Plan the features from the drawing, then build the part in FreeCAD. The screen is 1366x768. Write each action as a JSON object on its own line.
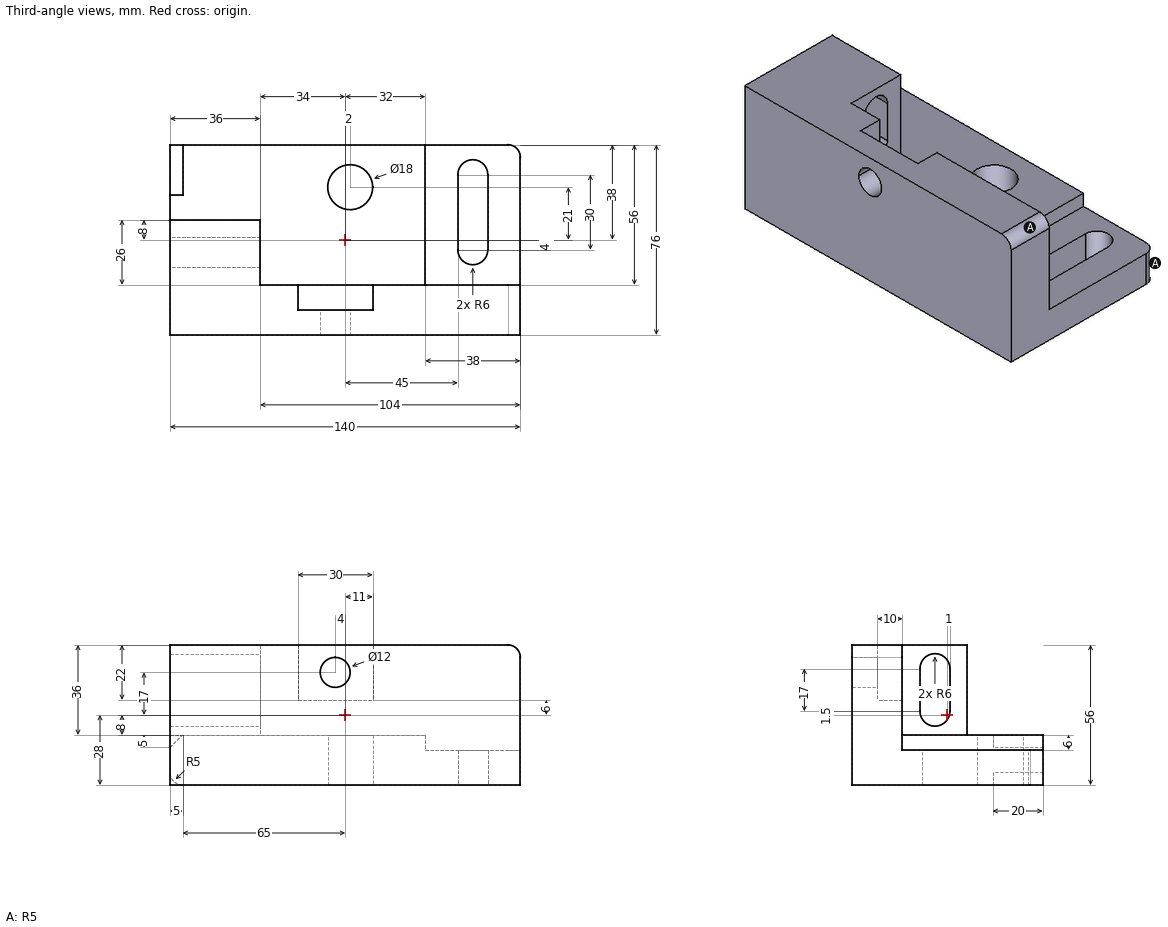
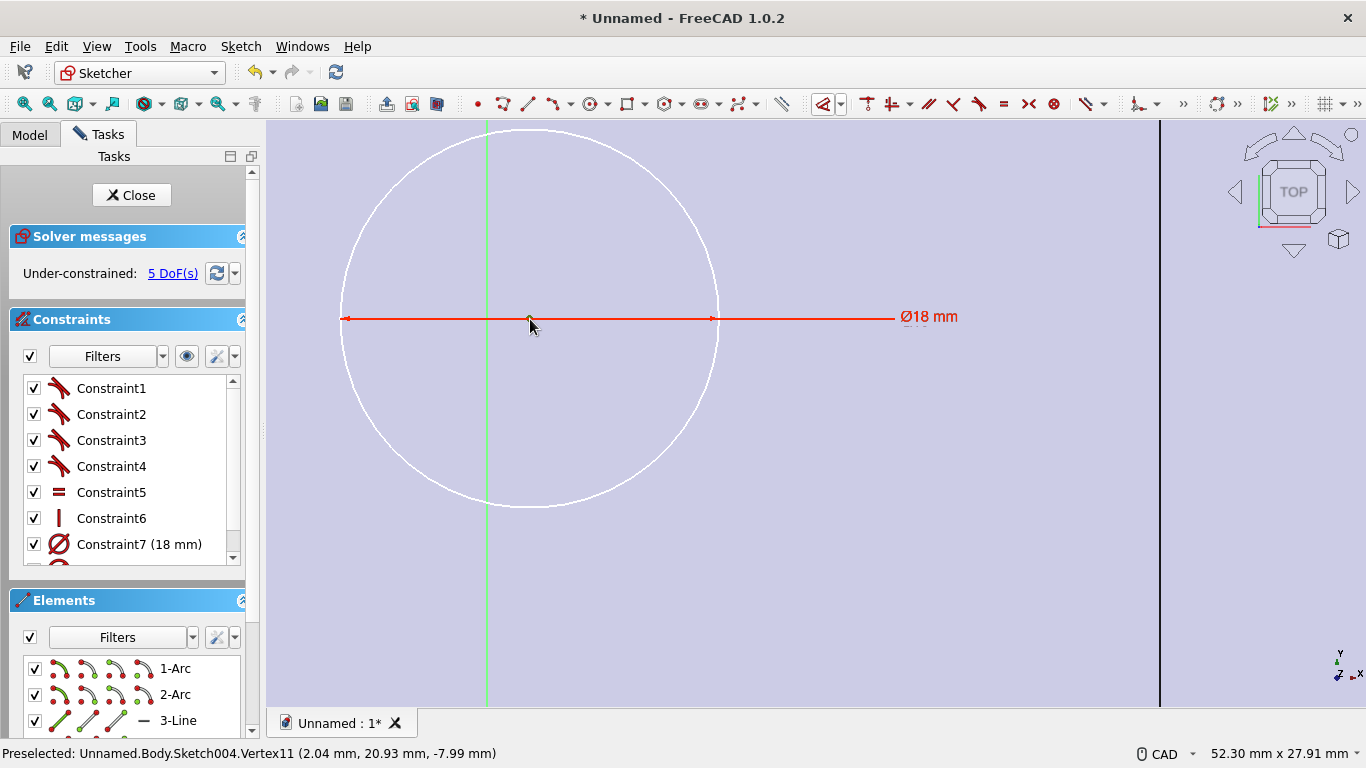
{"action": "key", "text": "l"}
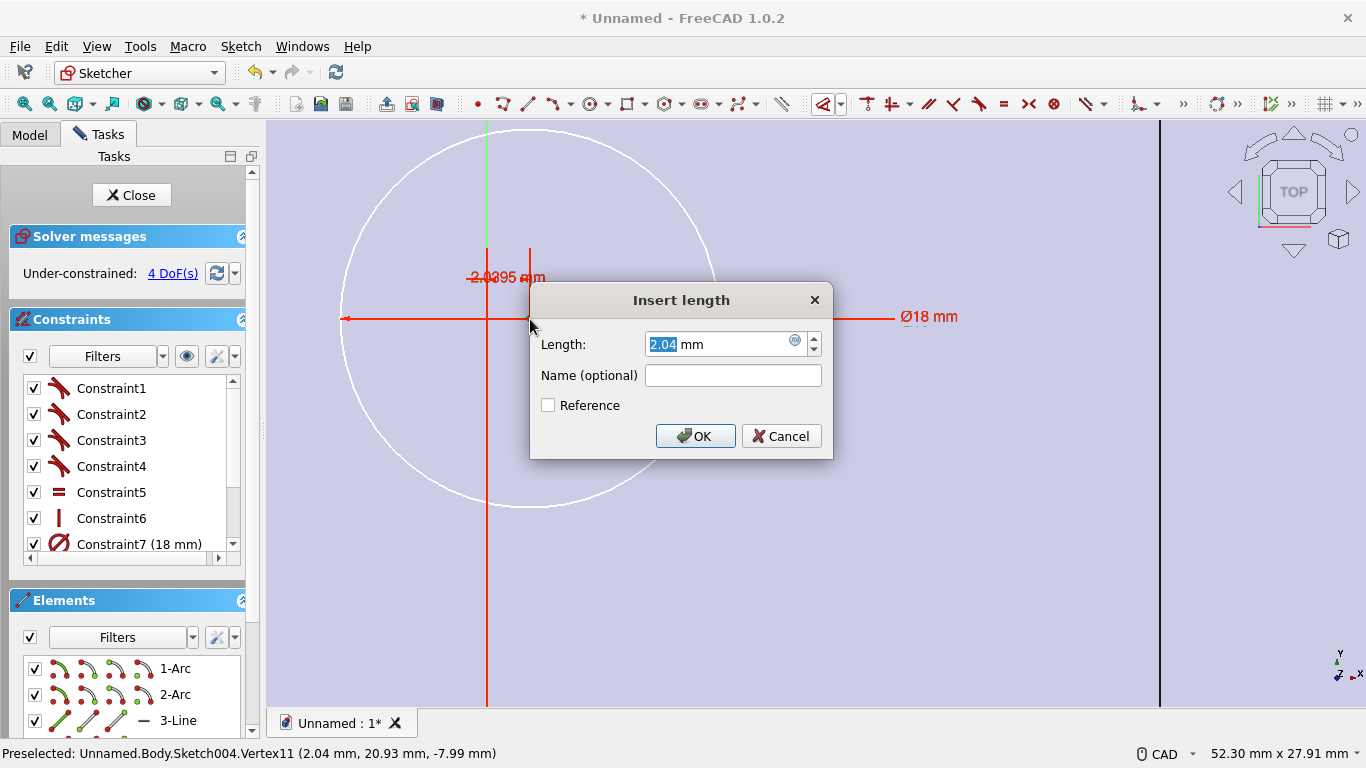
{"action": "type", "text": "2"}
{"action": "key", "text": "Return"}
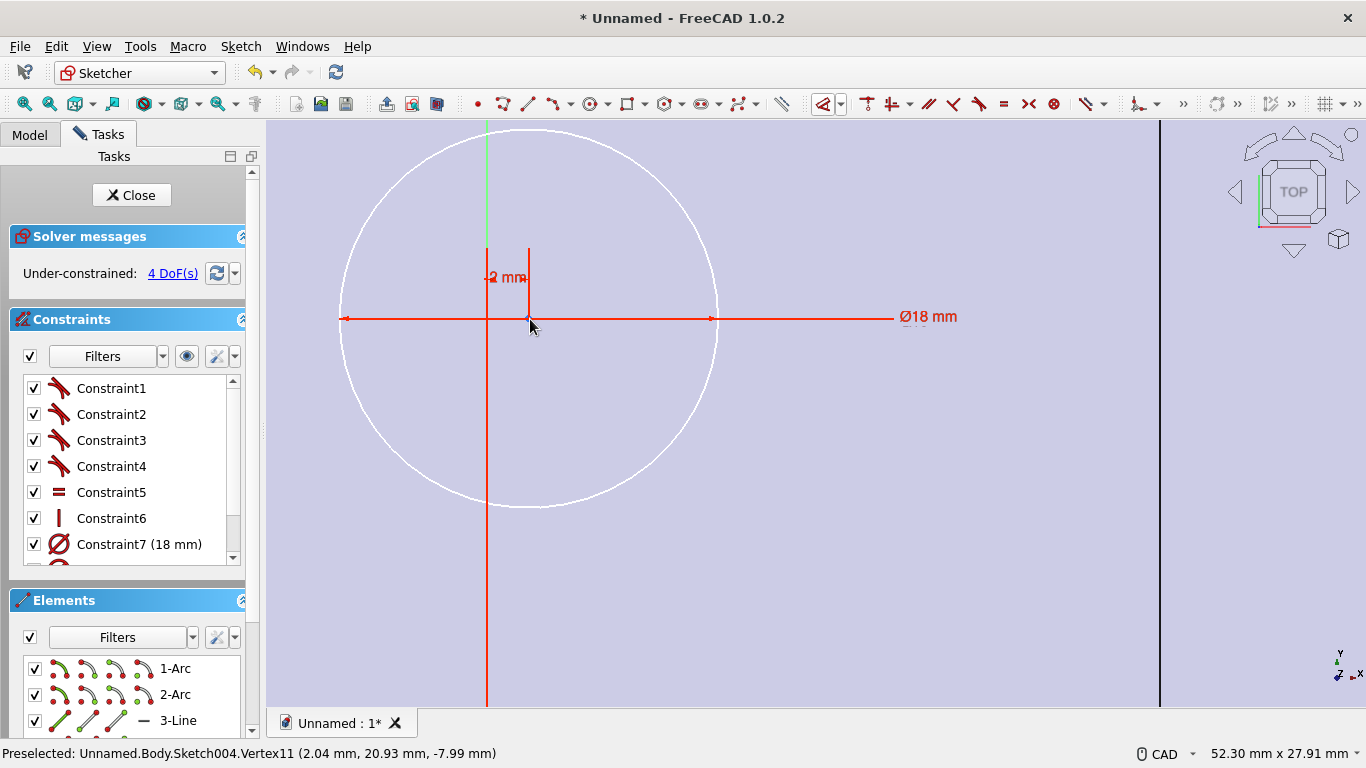
{"action": "scroll", "coordinate": [531, 321], "scroll_direction": "down", "scroll_amount": 4}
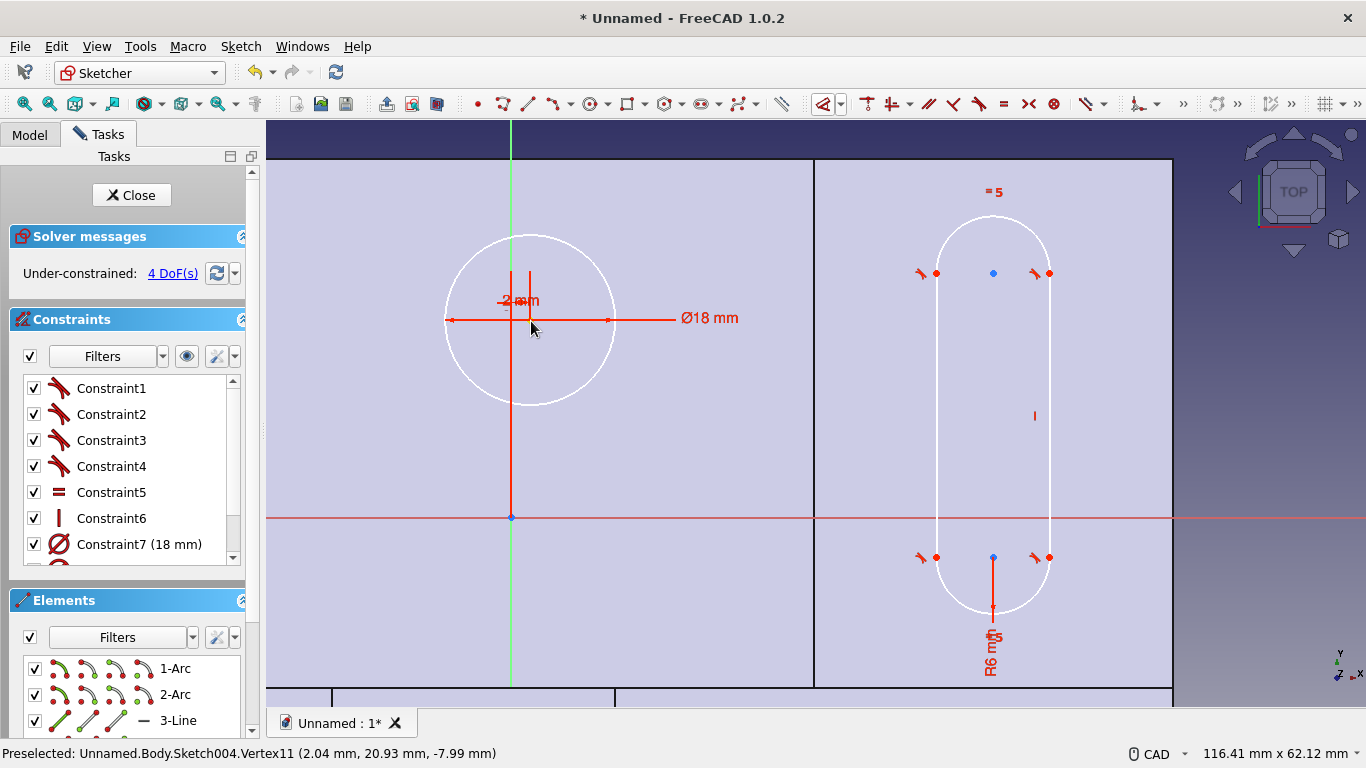
{"action": "left_click", "coordinate": [937, 472]}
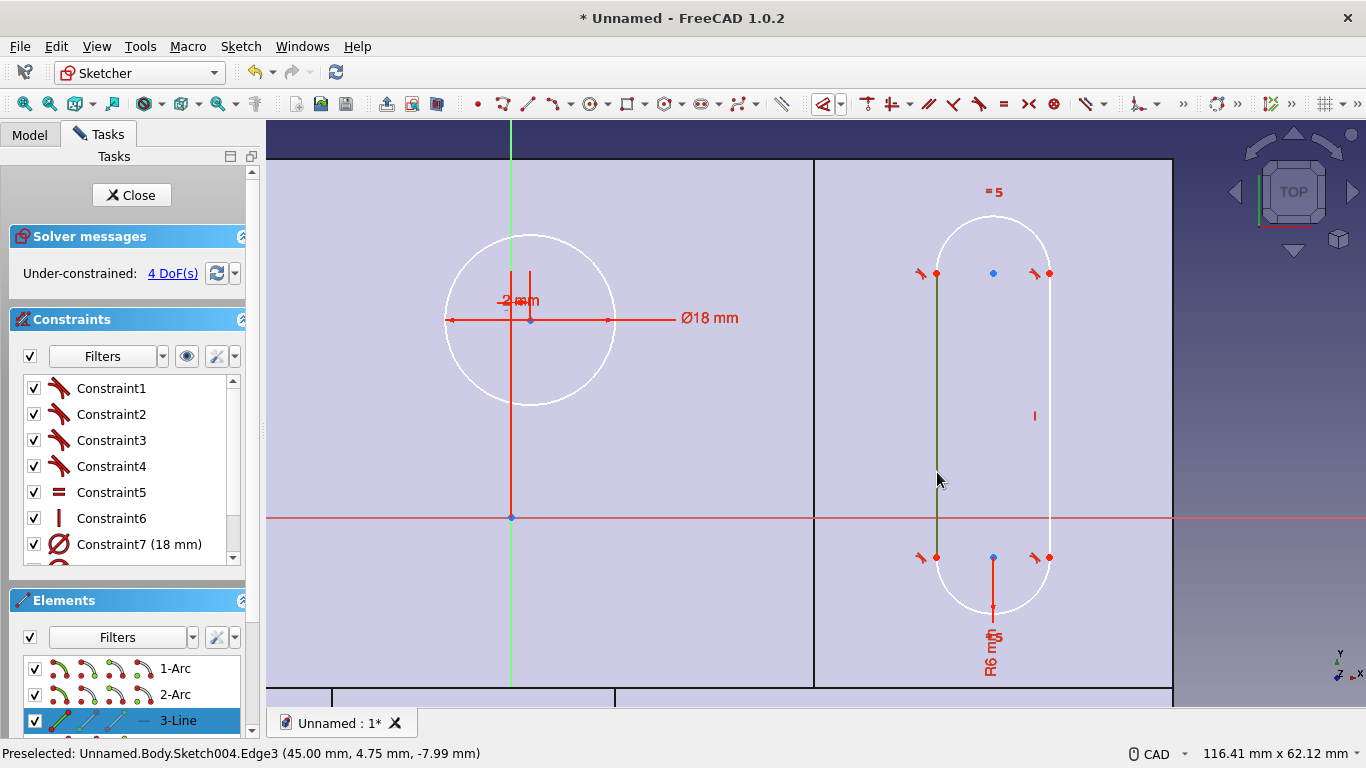
{"action": "left_click", "coordinate": [840, 104]}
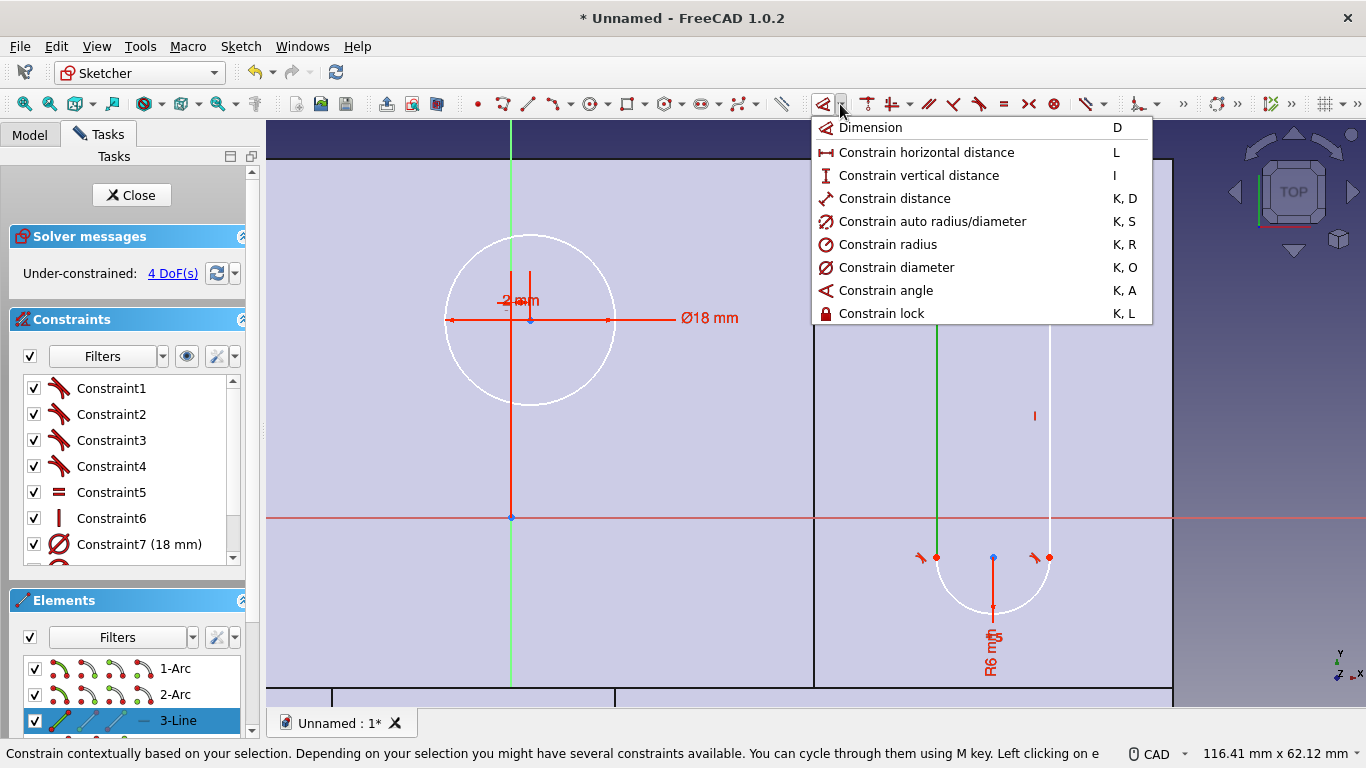
{"action": "left_click", "coordinate": [982, 176]}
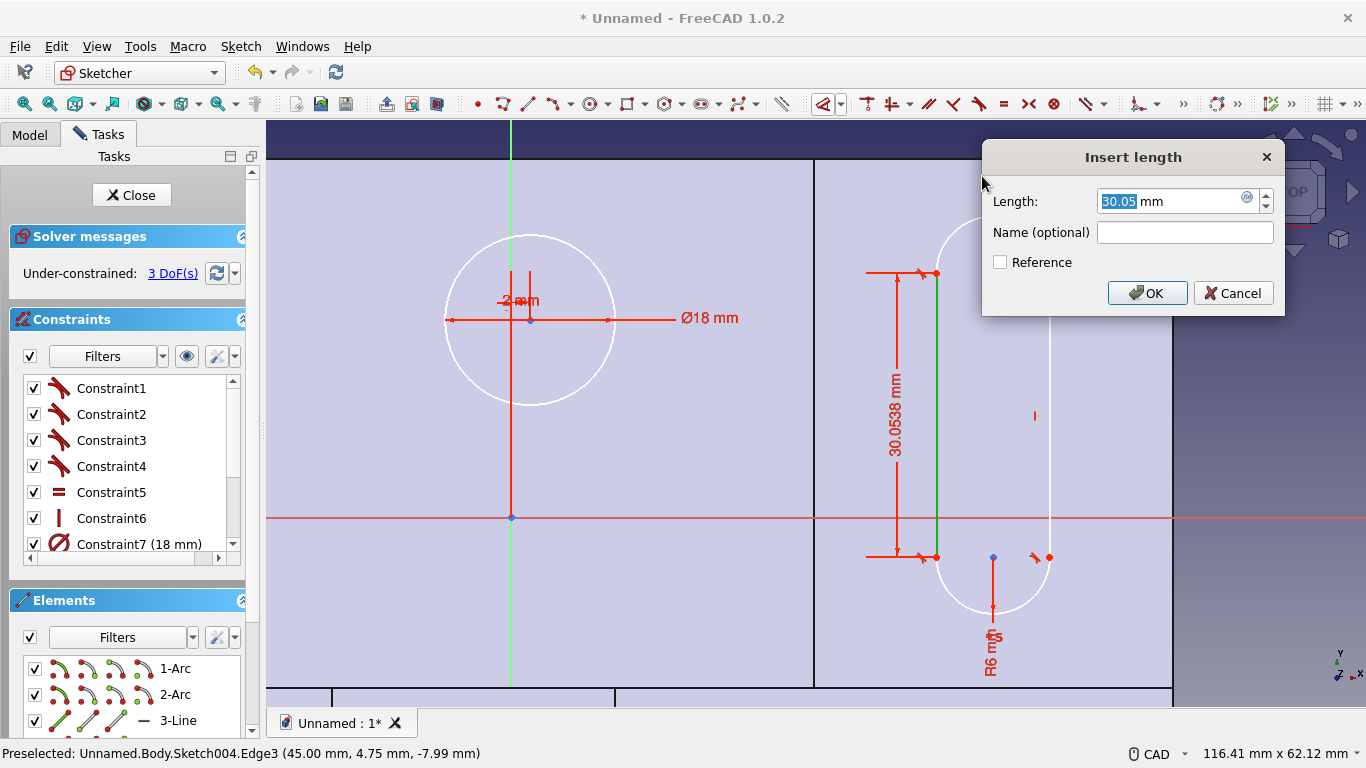
{"action": "type", "text": "30"}
{"action": "key", "text": "Return"}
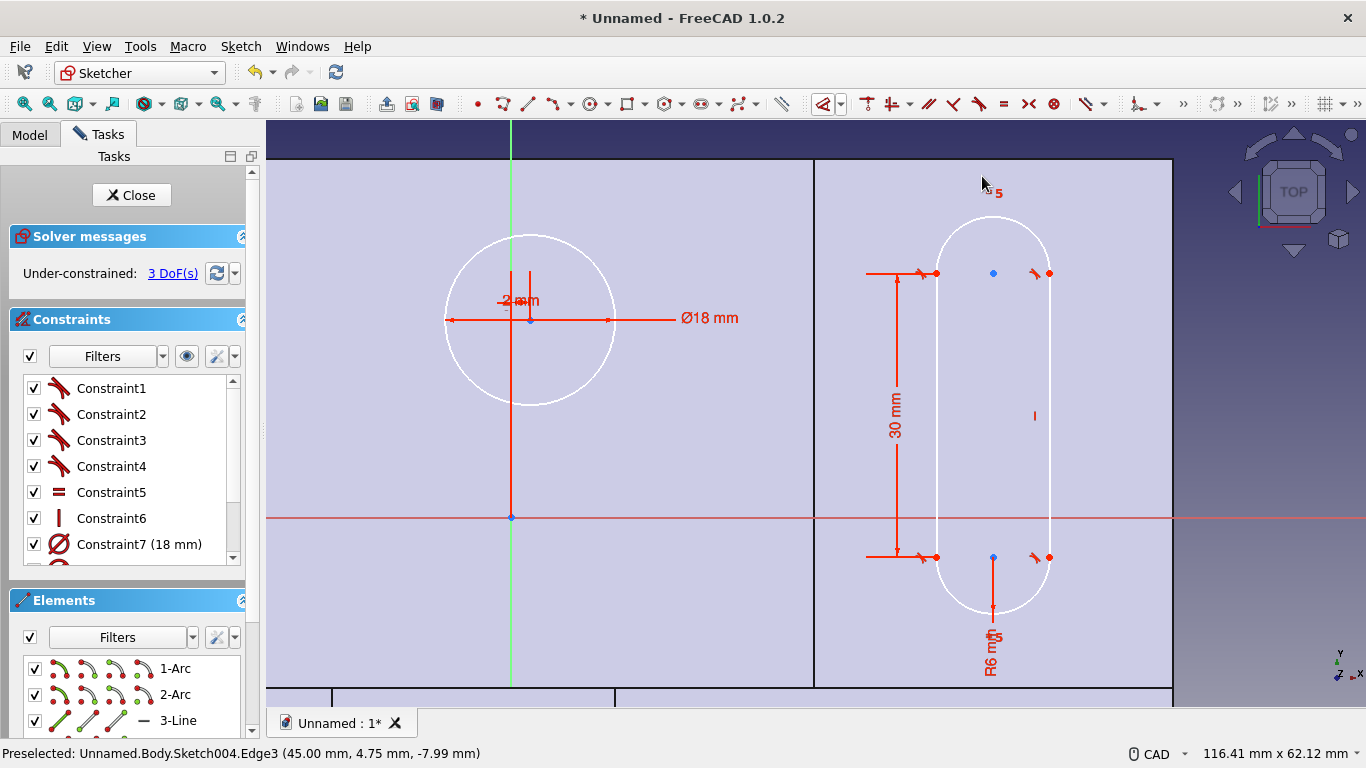
{"action": "left_click", "coordinate": [937, 557]}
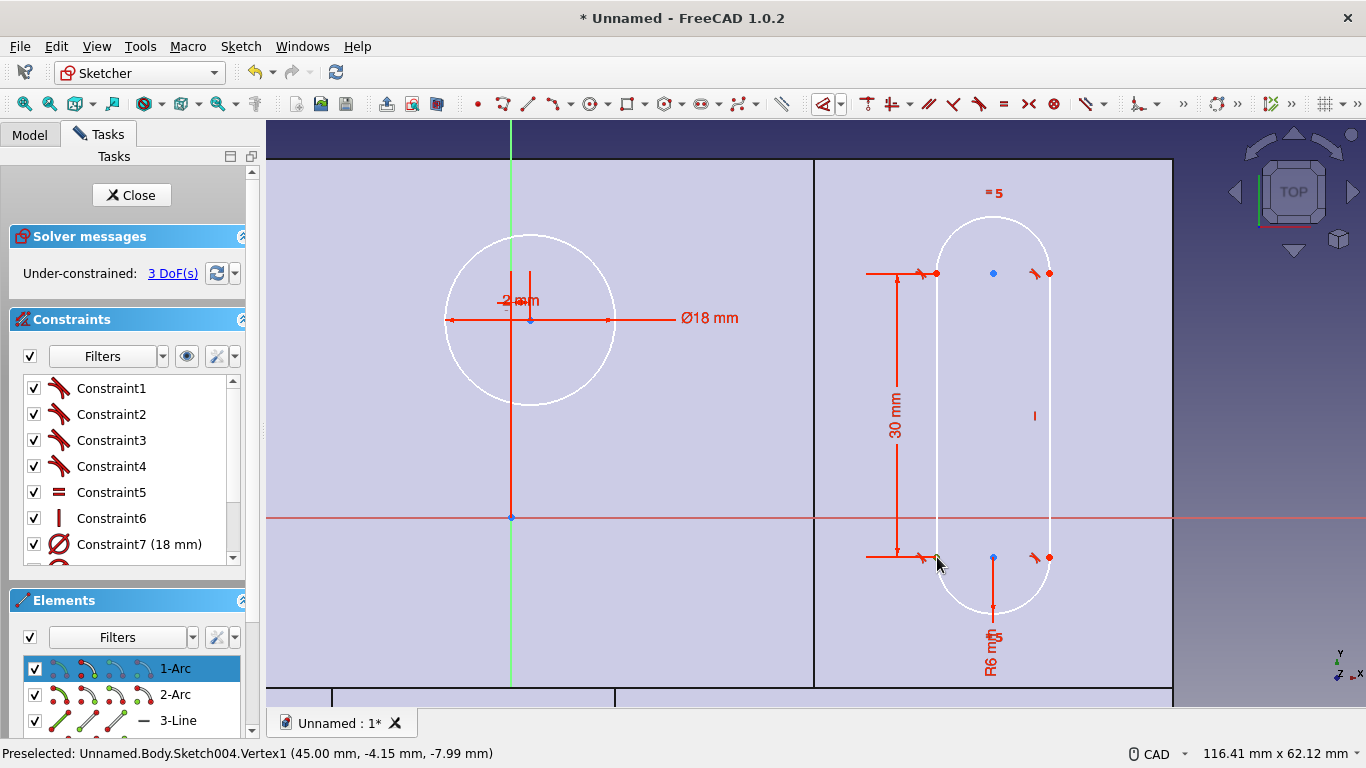
{"action": "key", "text": "i"}